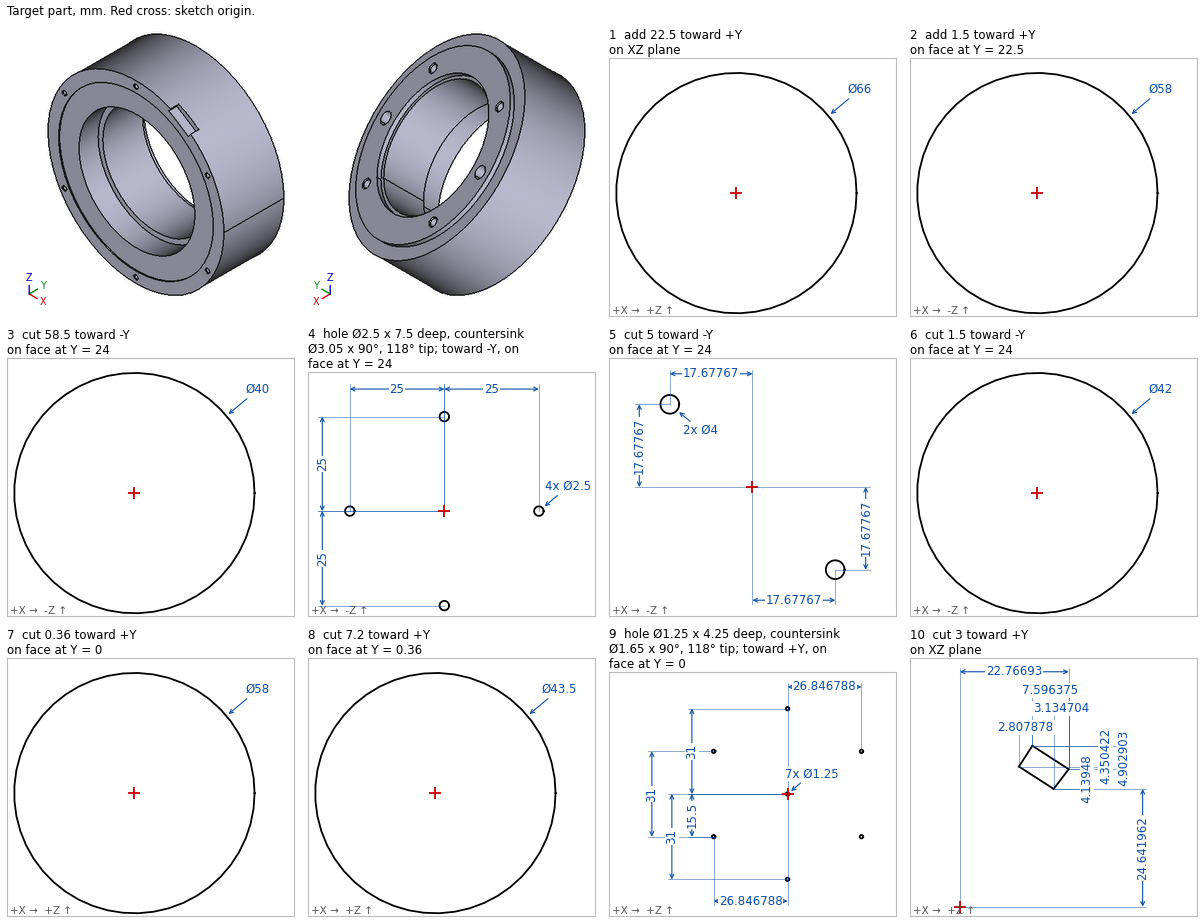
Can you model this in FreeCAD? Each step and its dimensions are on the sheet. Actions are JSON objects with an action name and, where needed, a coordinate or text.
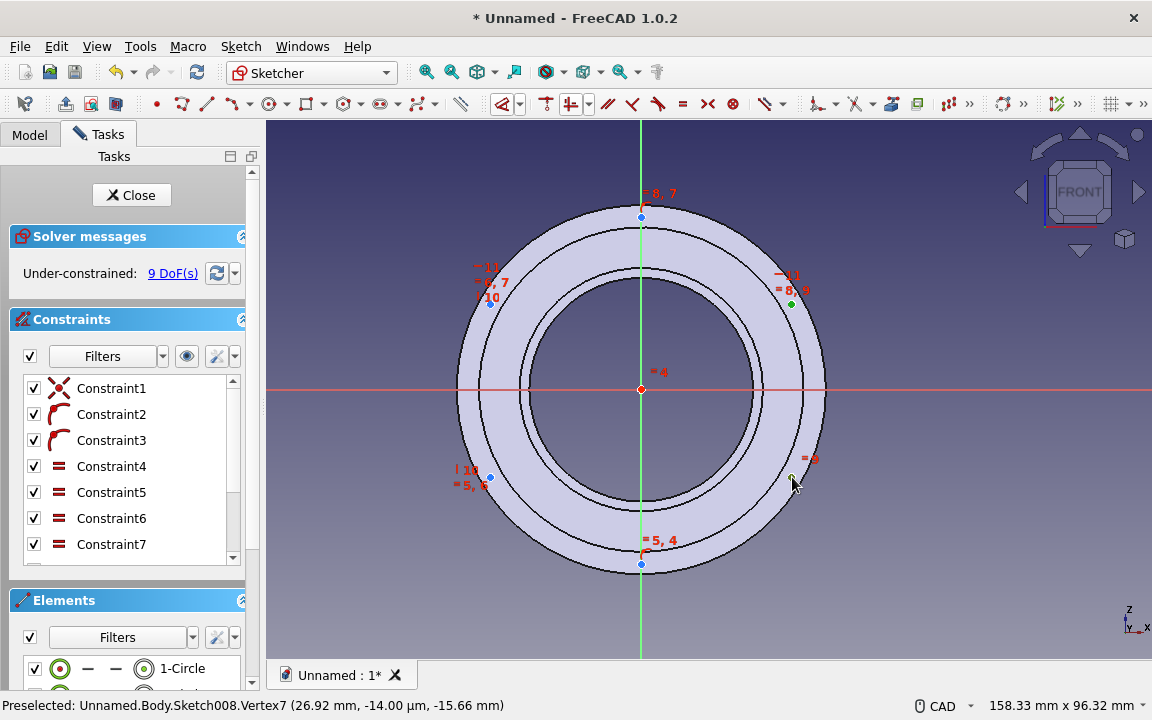
{"action": "key", "text": "v"}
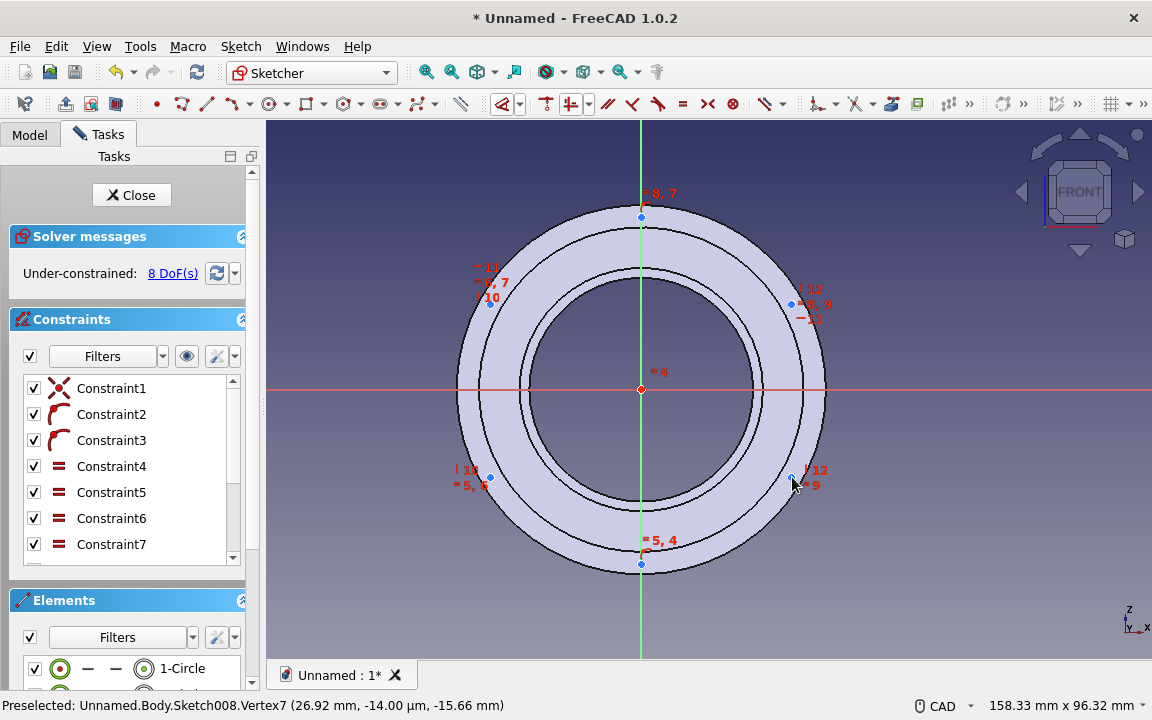
{"action": "left_click", "coordinate": [491, 477]}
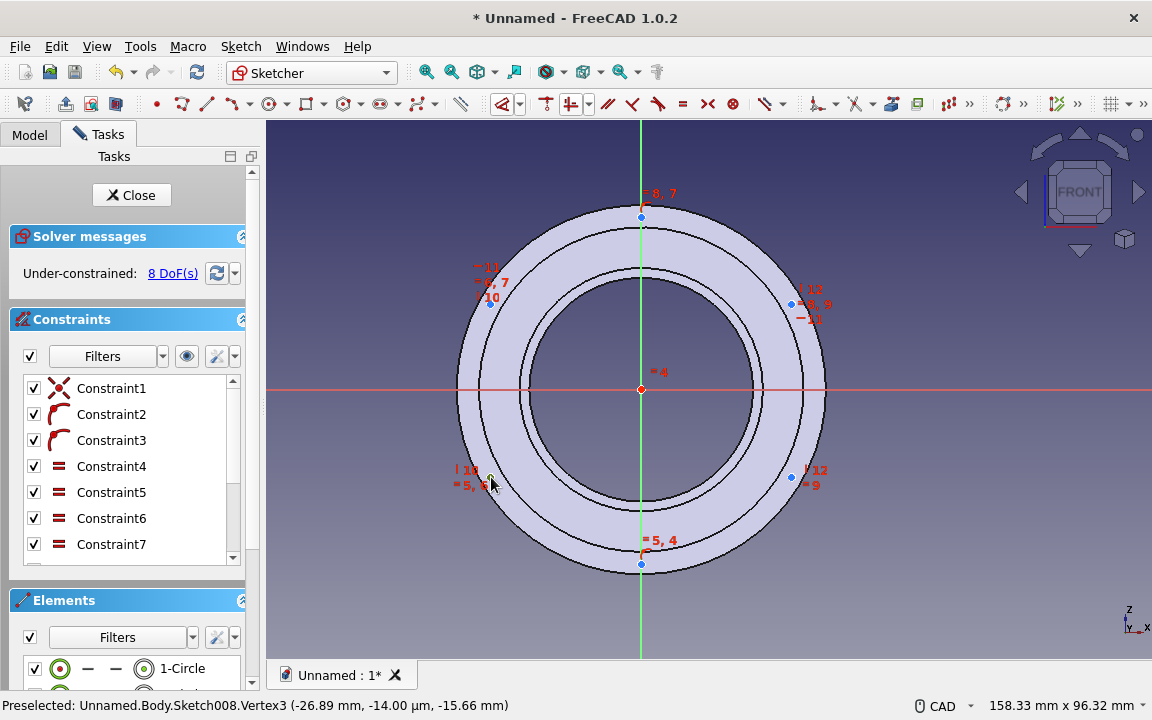
{"action": "left_click", "coordinate": [792, 477]}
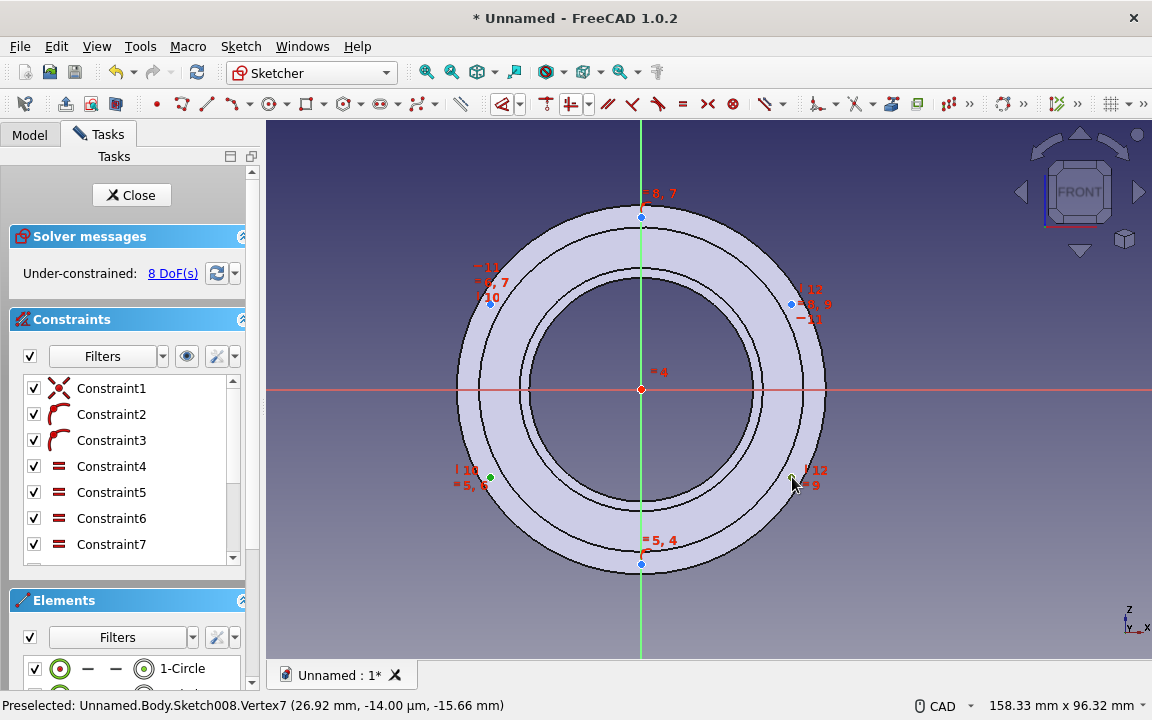
{"action": "key", "text": "h"}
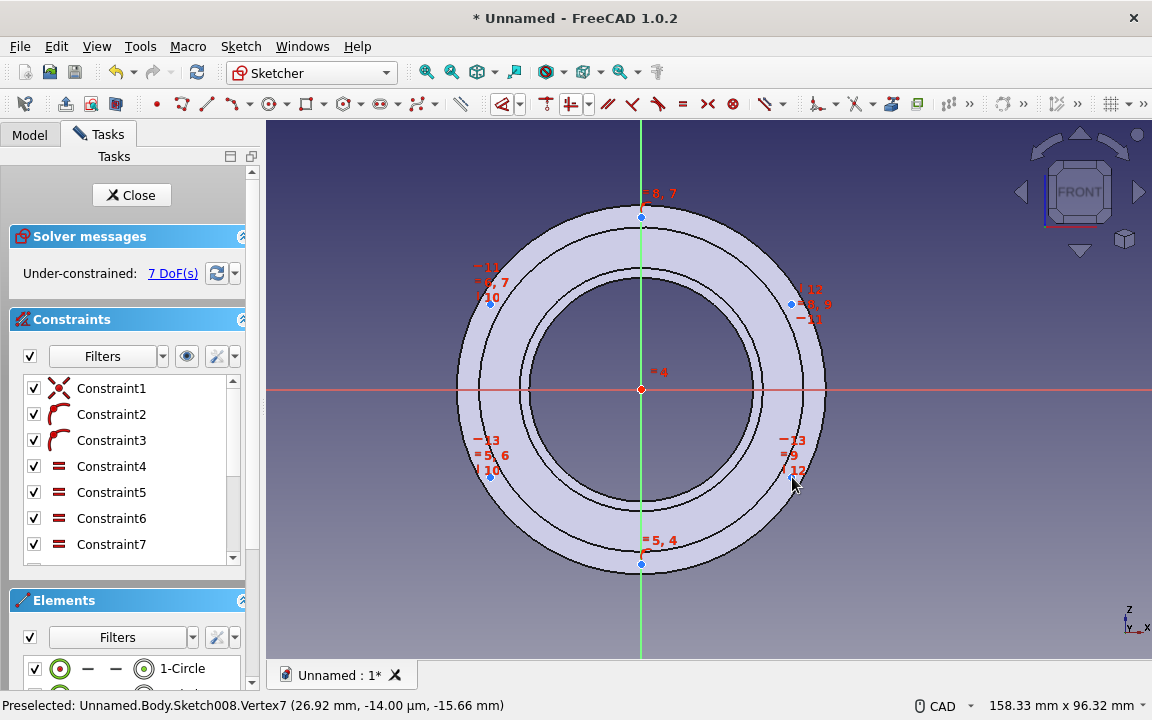
{"action": "scroll", "coordinate": [644, 387], "scroll_direction": "up", "scroll_amount": 9}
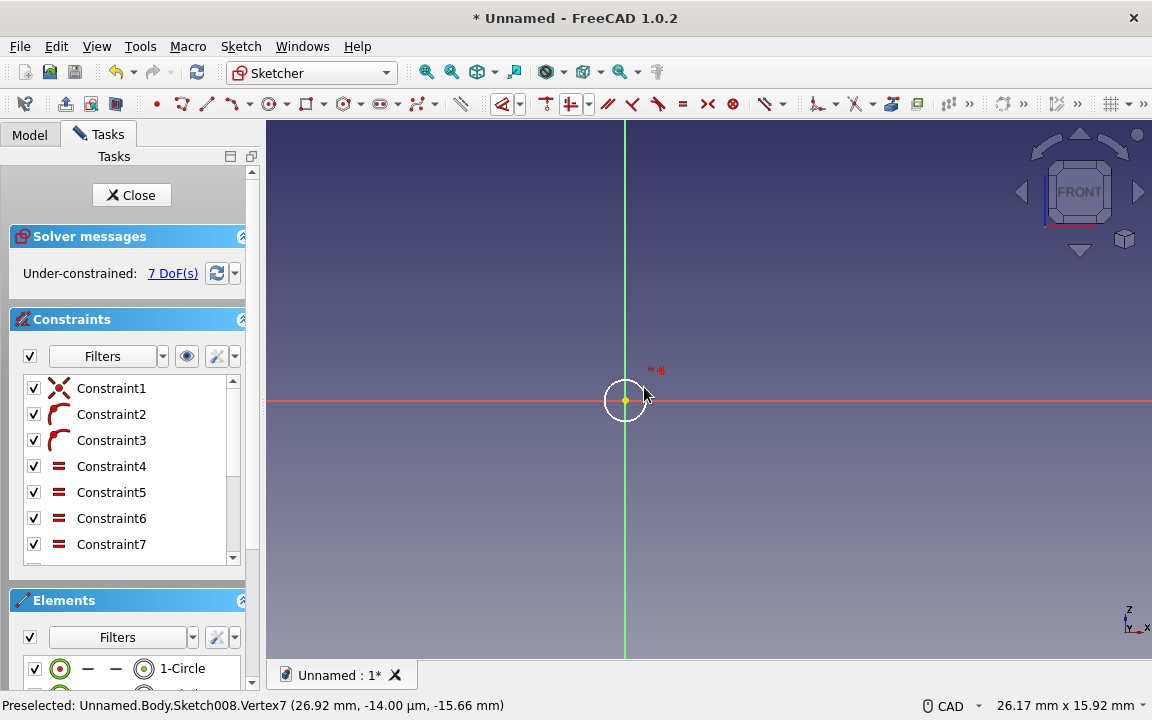
{"action": "left_click", "coordinate": [640, 386]}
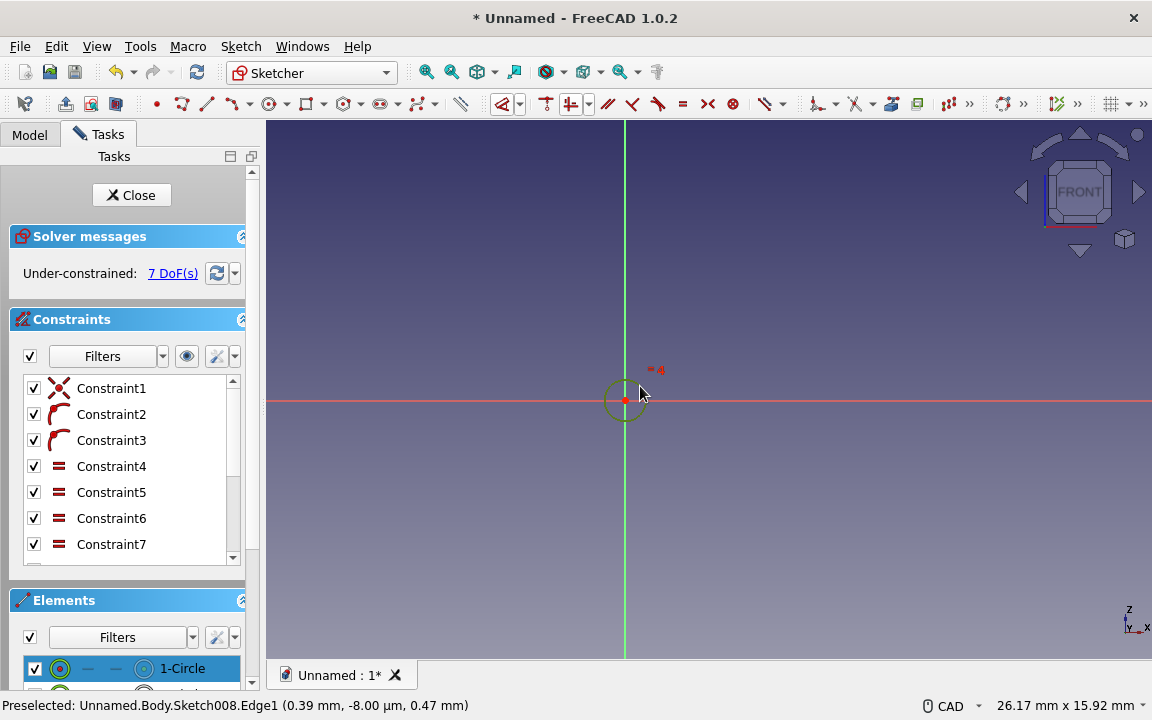
{"action": "key", "text": "k o"}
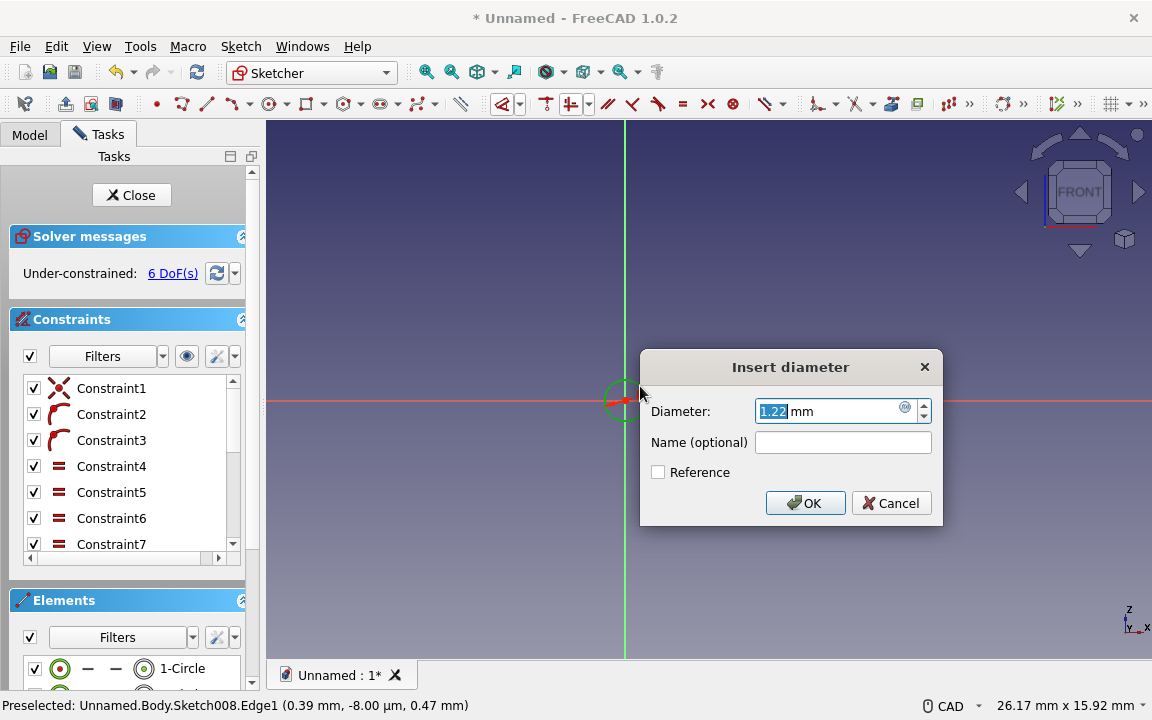
{"action": "type", "text": "1.25"}
{"action": "key", "text": "Return"}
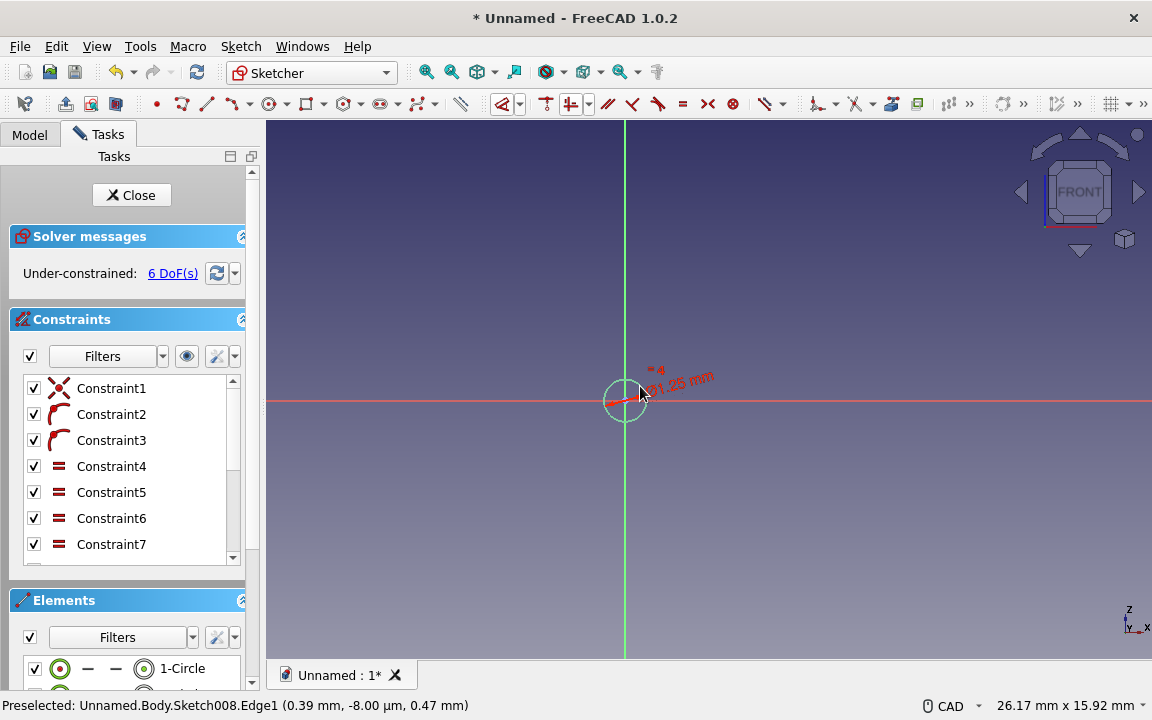
{"action": "scroll", "coordinate": [644, 387], "scroll_direction": "down", "scroll_amount": 9}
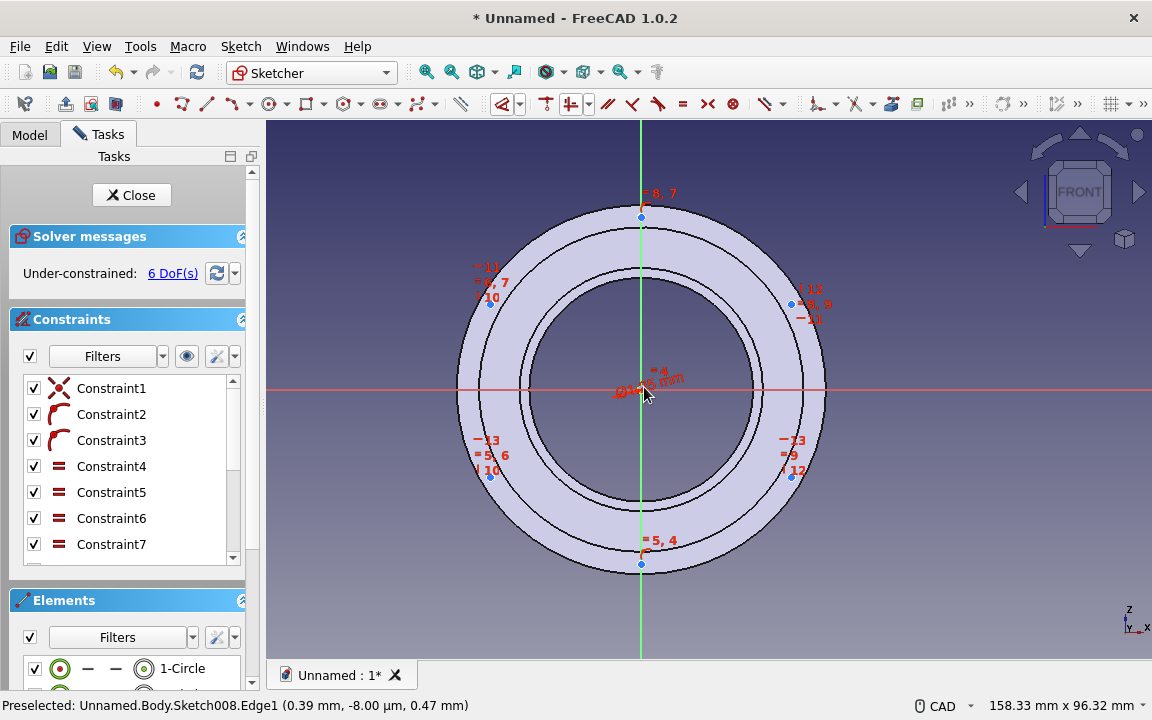
{"action": "left_click", "coordinate": [641, 564]}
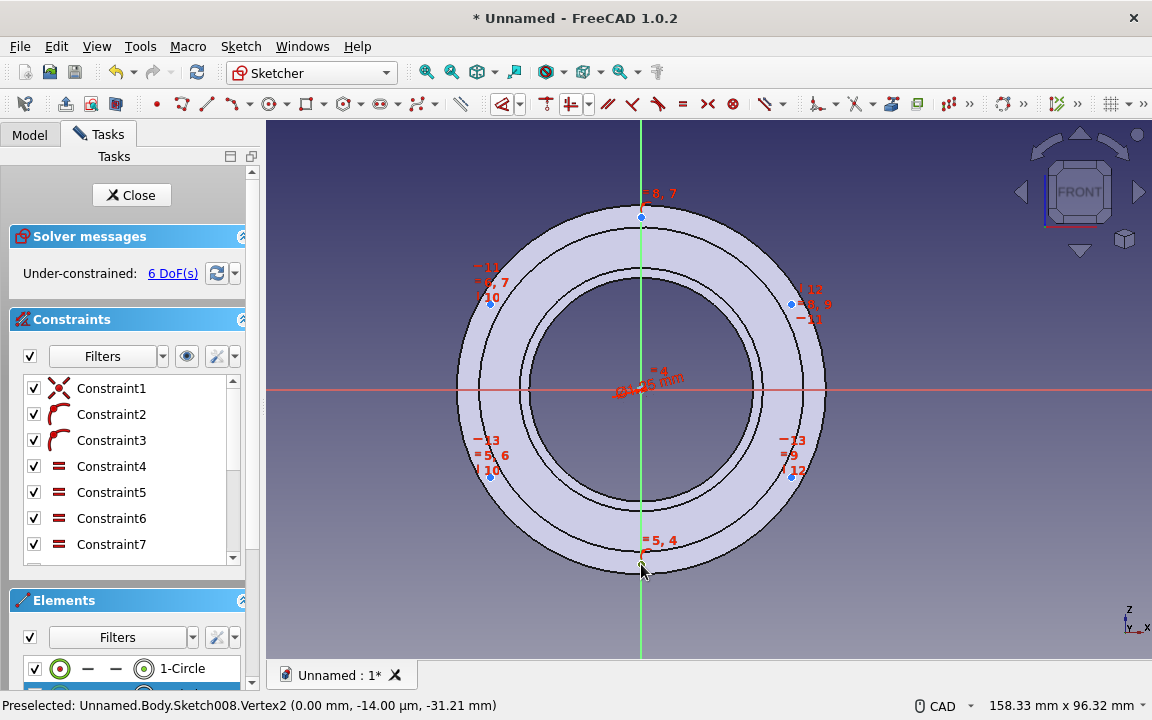
{"action": "key", "text": "i"}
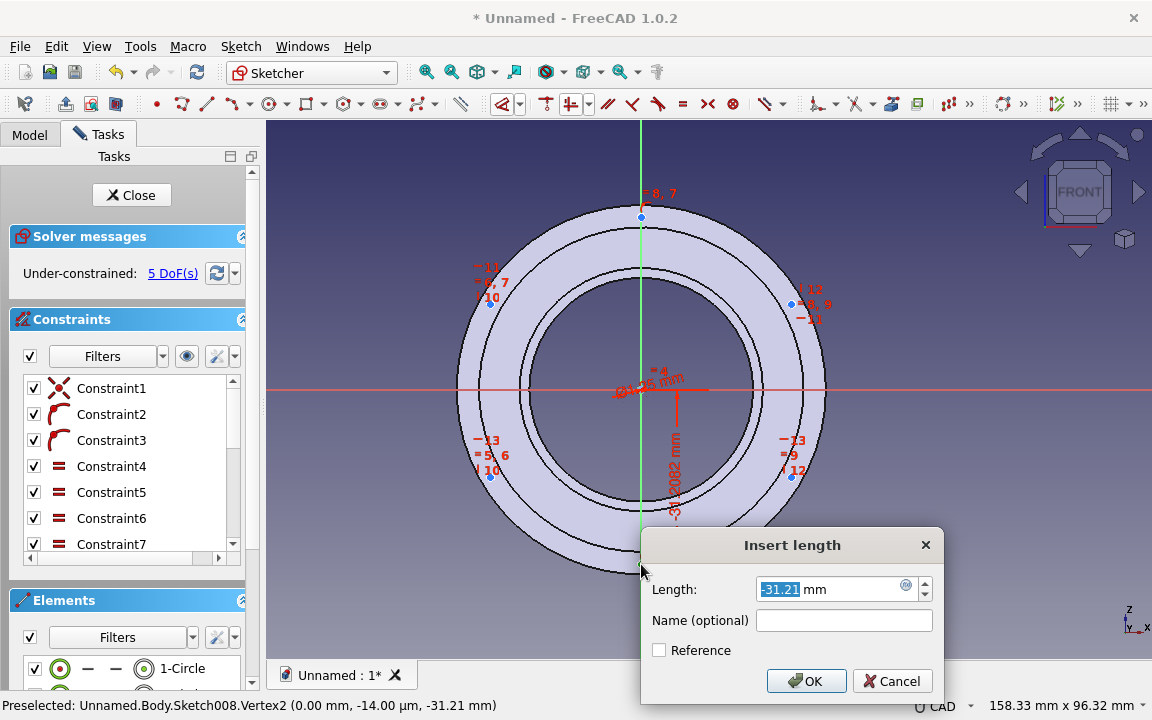
{"action": "type", "text": "-31"}
{"action": "key", "text": "Return"}